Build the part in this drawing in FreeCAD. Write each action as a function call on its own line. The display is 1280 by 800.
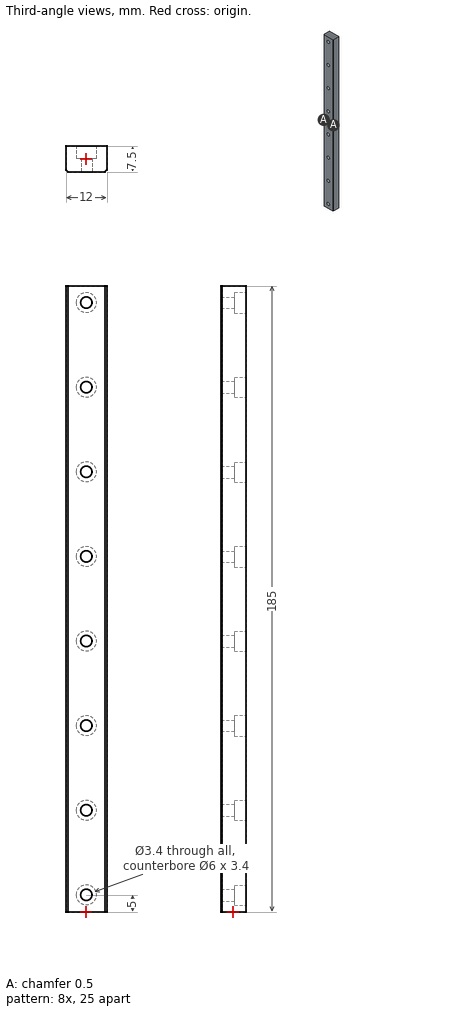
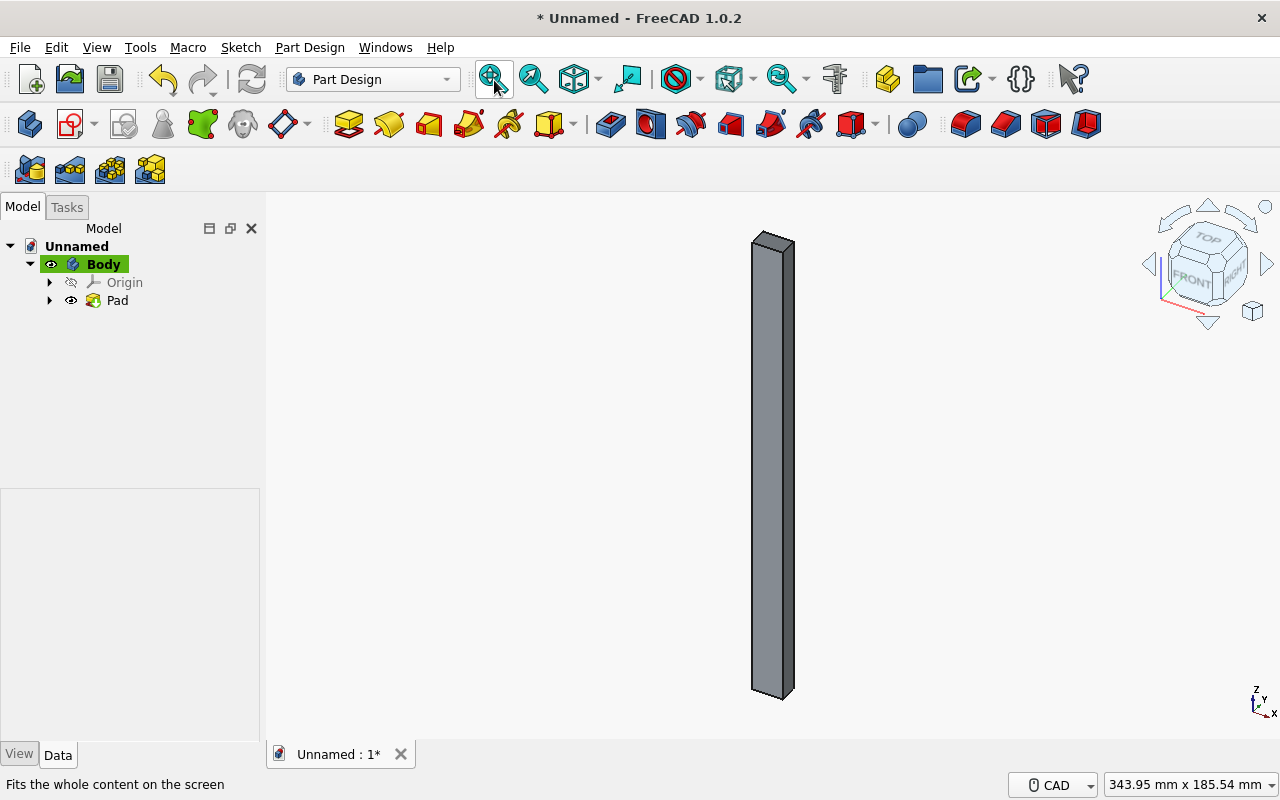
click(783, 475)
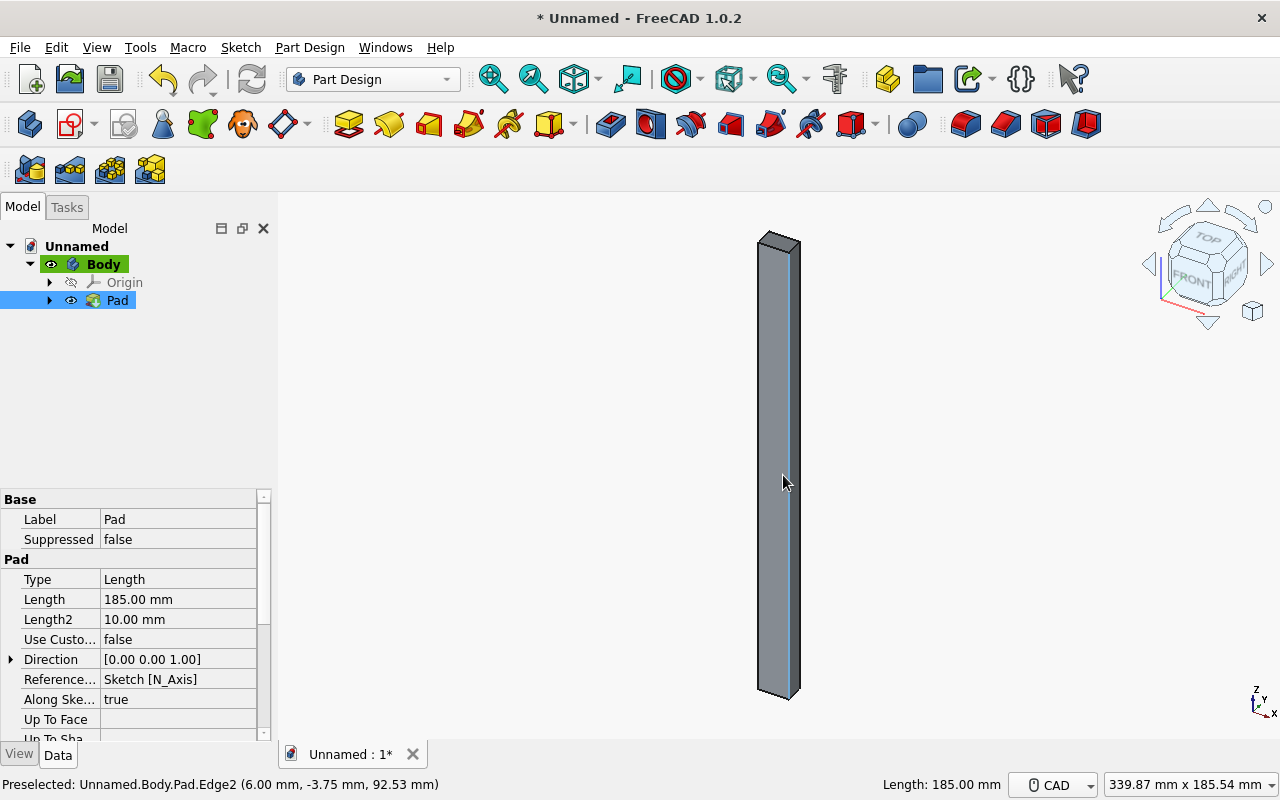
key(0)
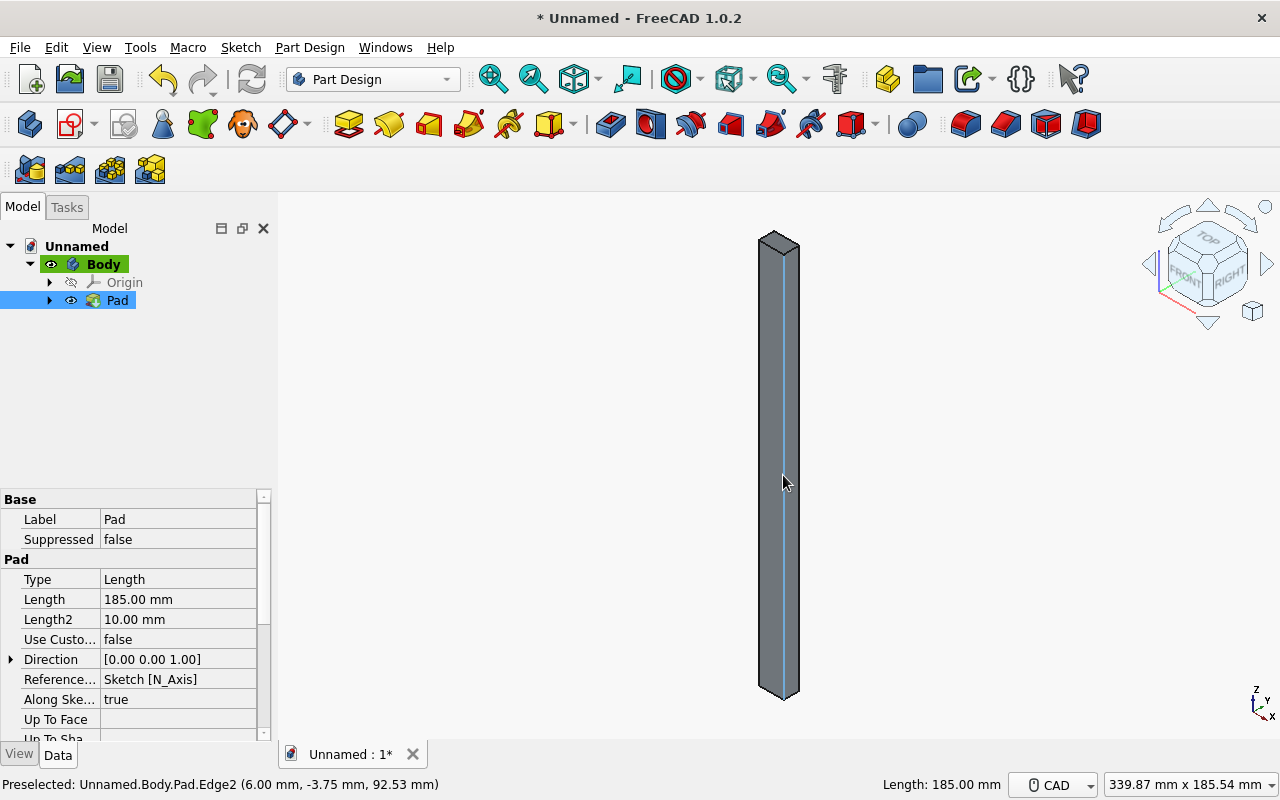
key(2)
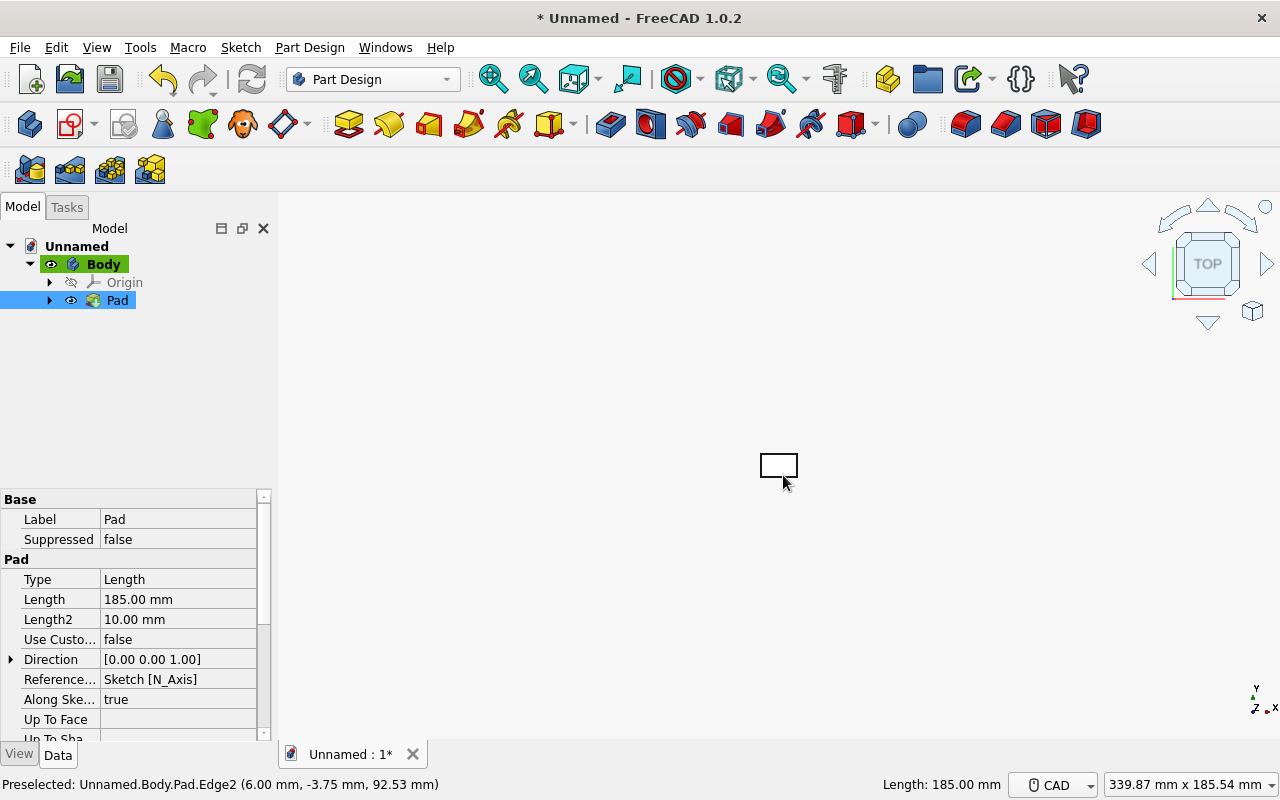
click(494, 80)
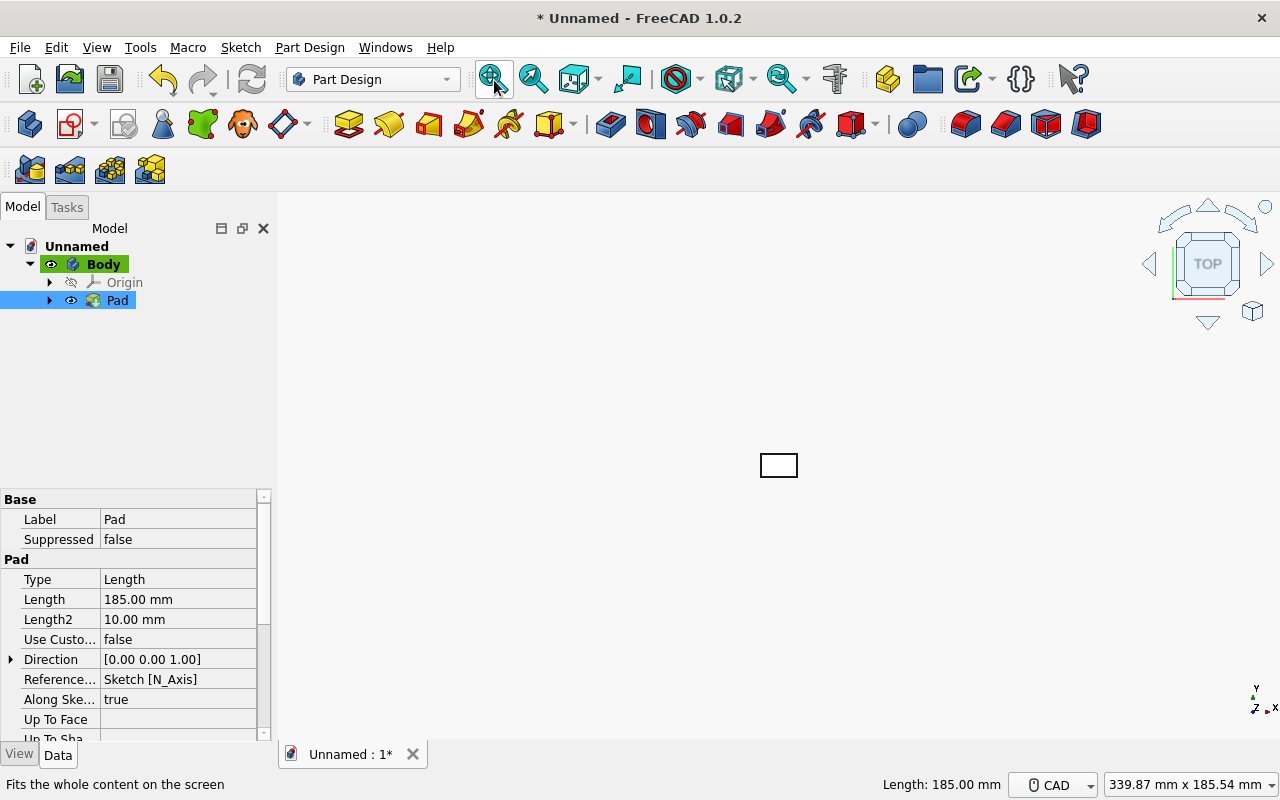
key(1)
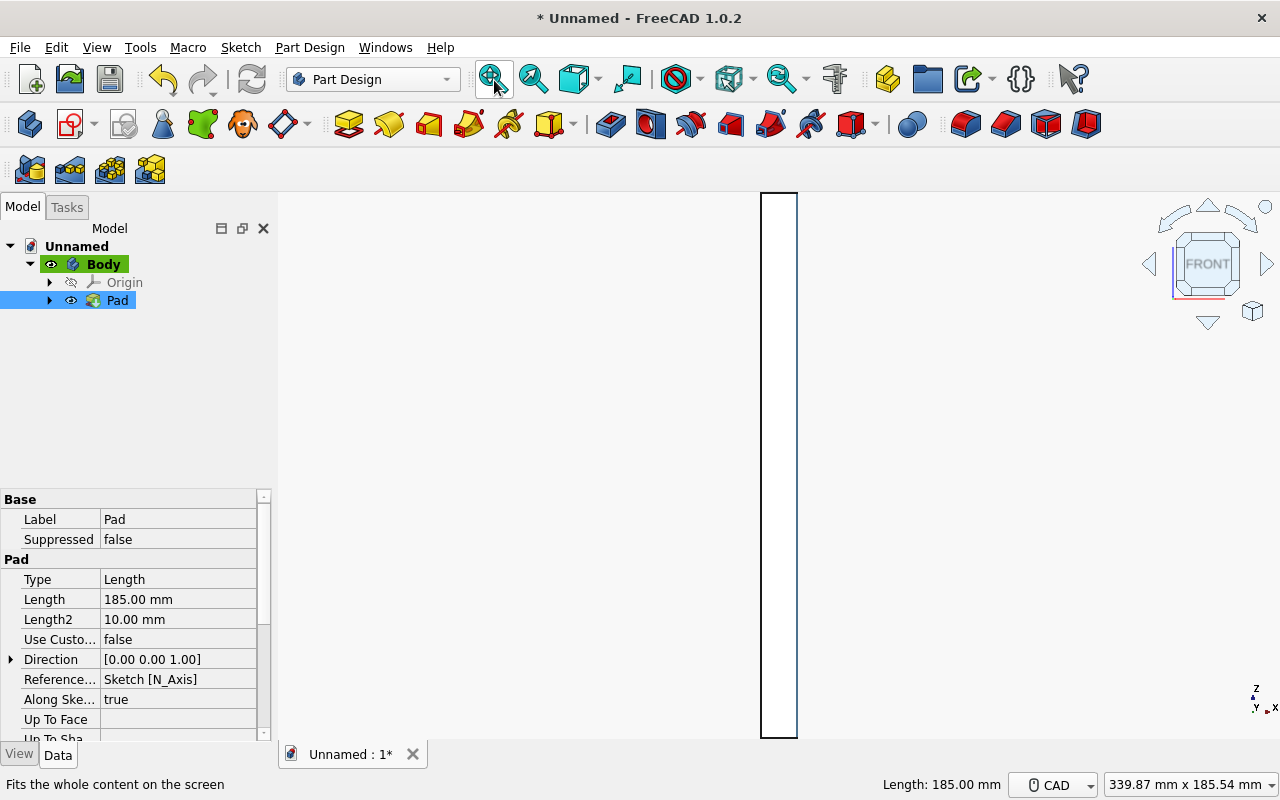
click(761, 464, ctrl)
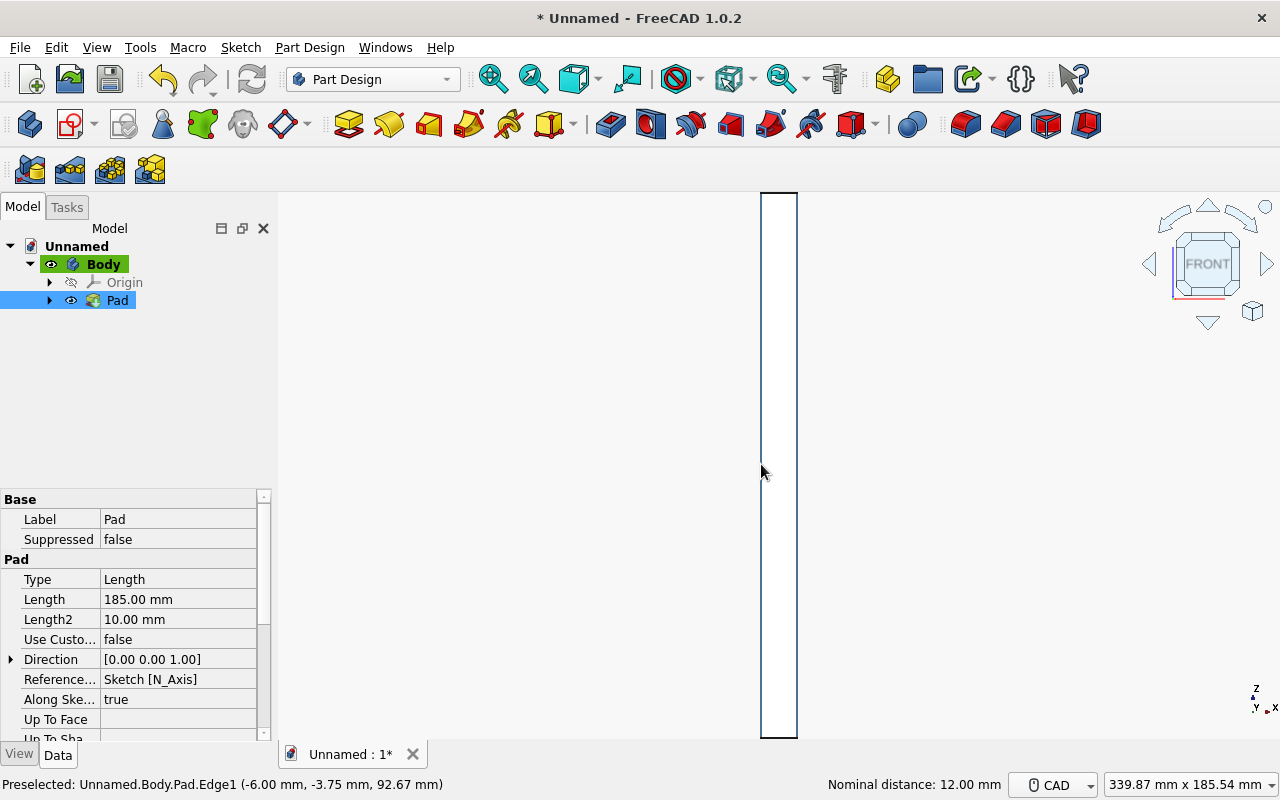
click(1006, 124)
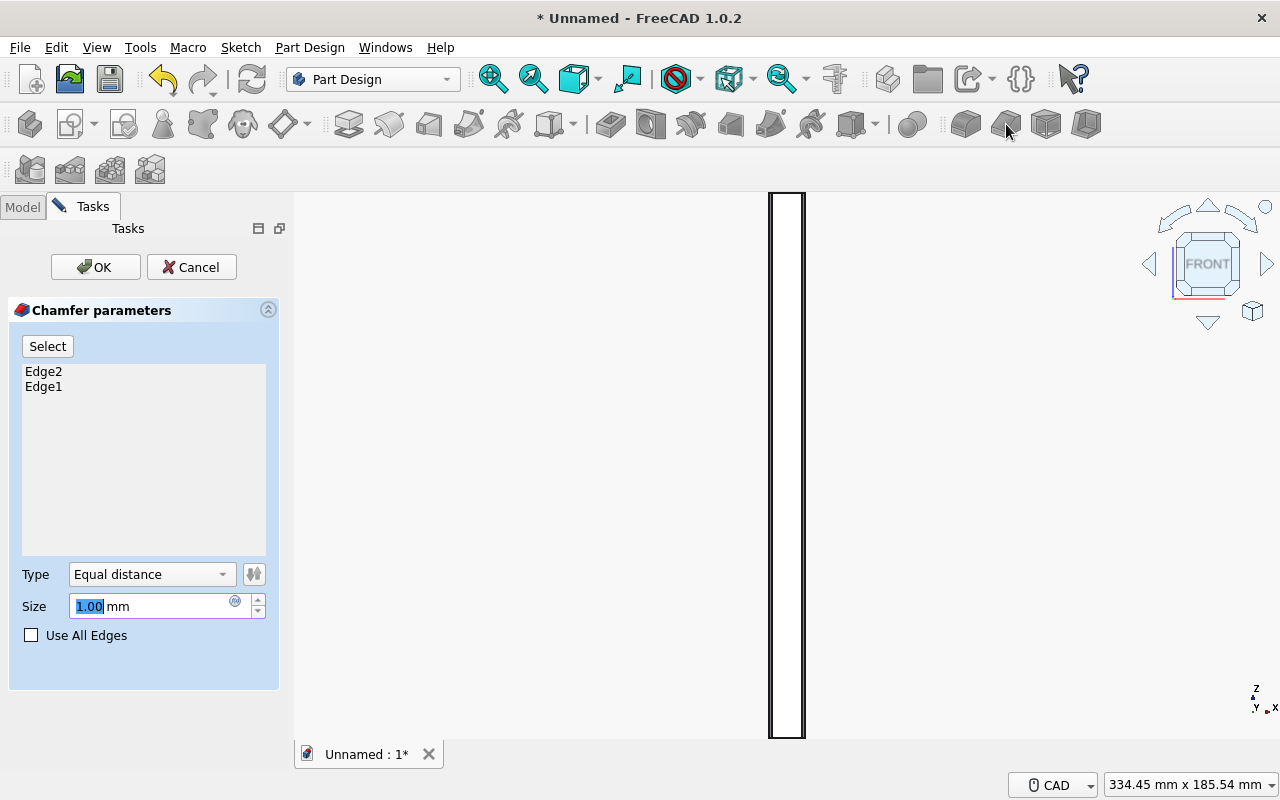
text(0.5)
key(Tab)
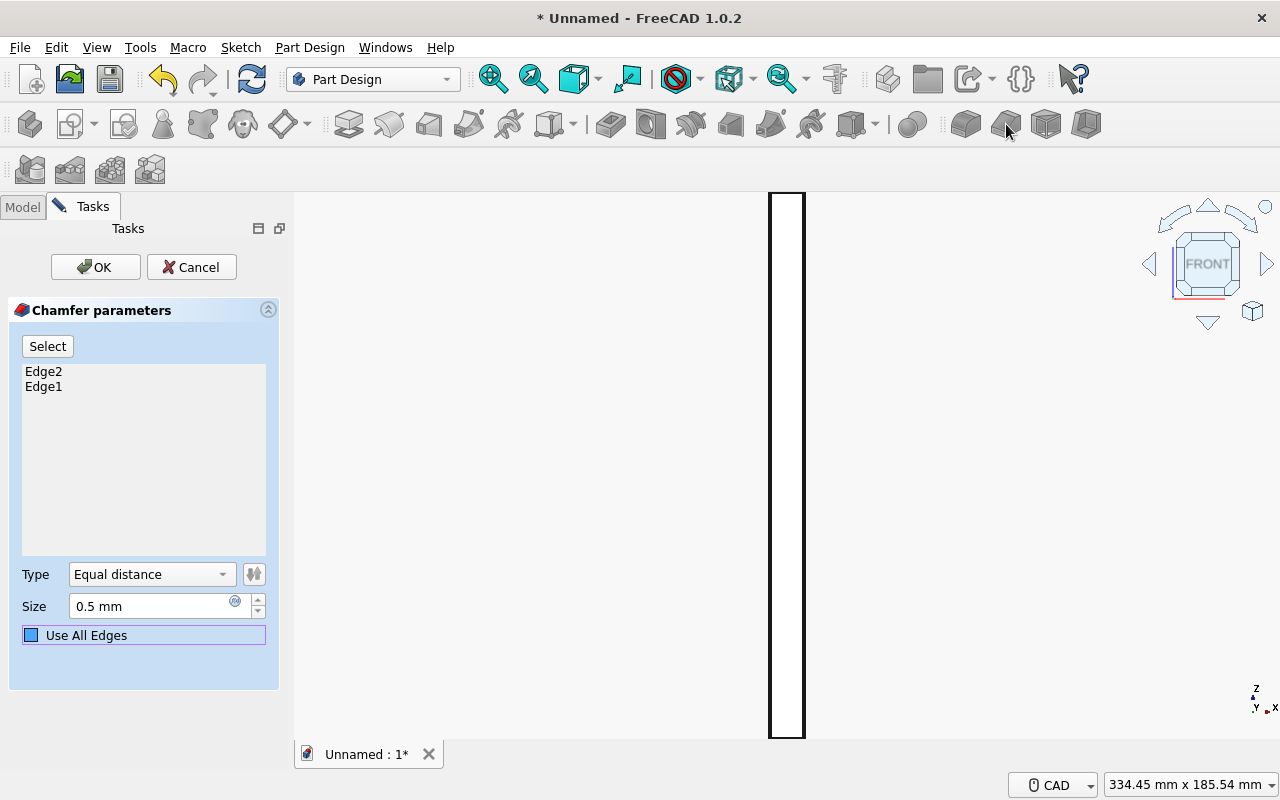
click(96, 267)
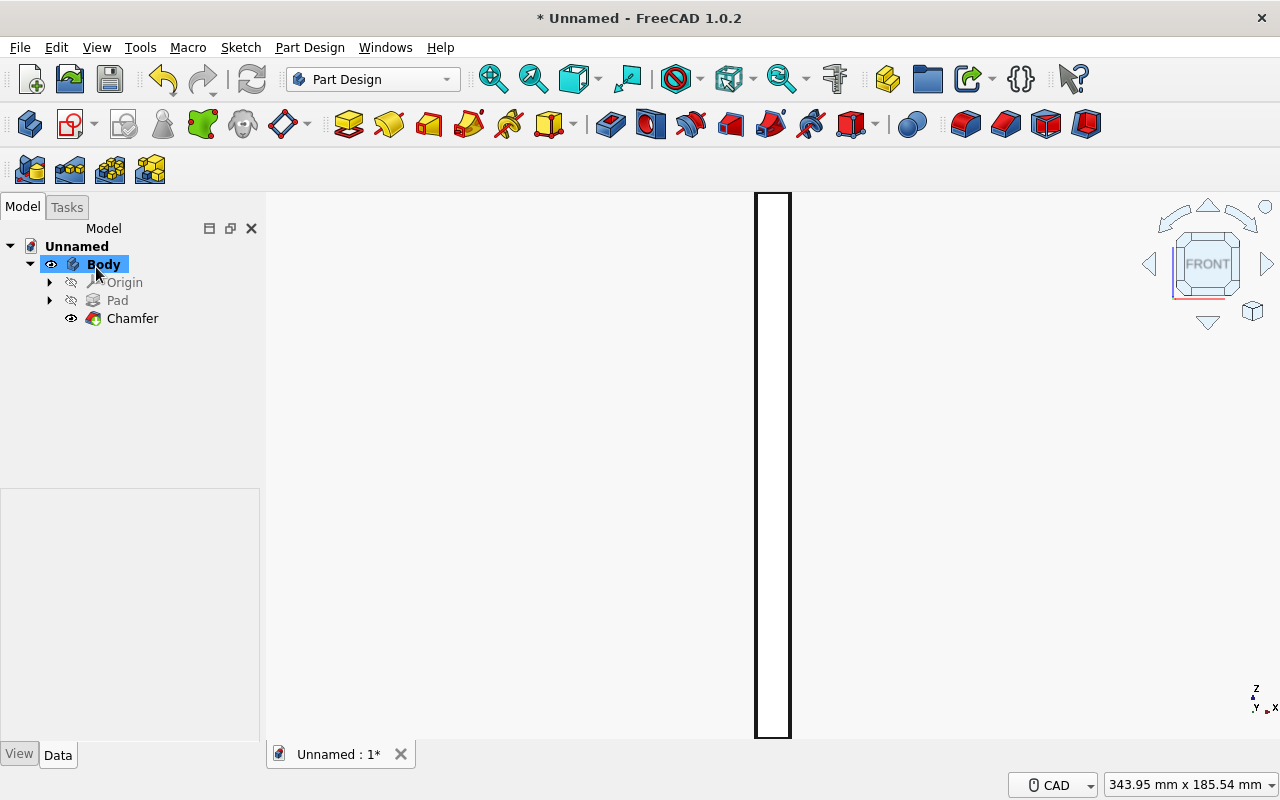
key(4)